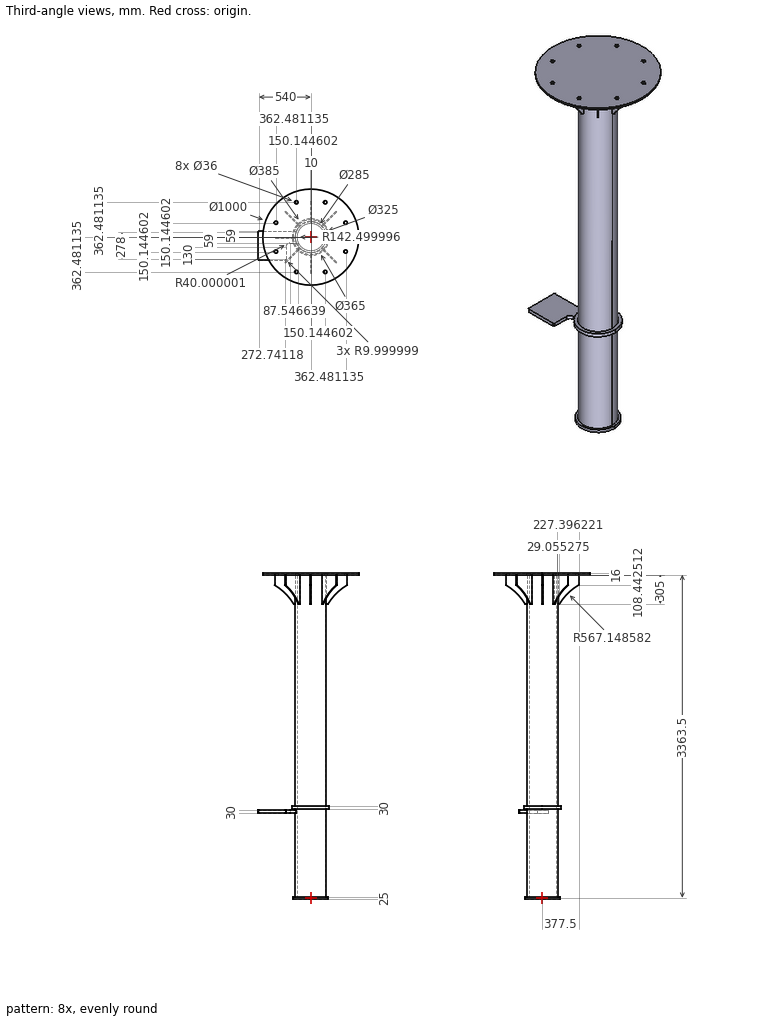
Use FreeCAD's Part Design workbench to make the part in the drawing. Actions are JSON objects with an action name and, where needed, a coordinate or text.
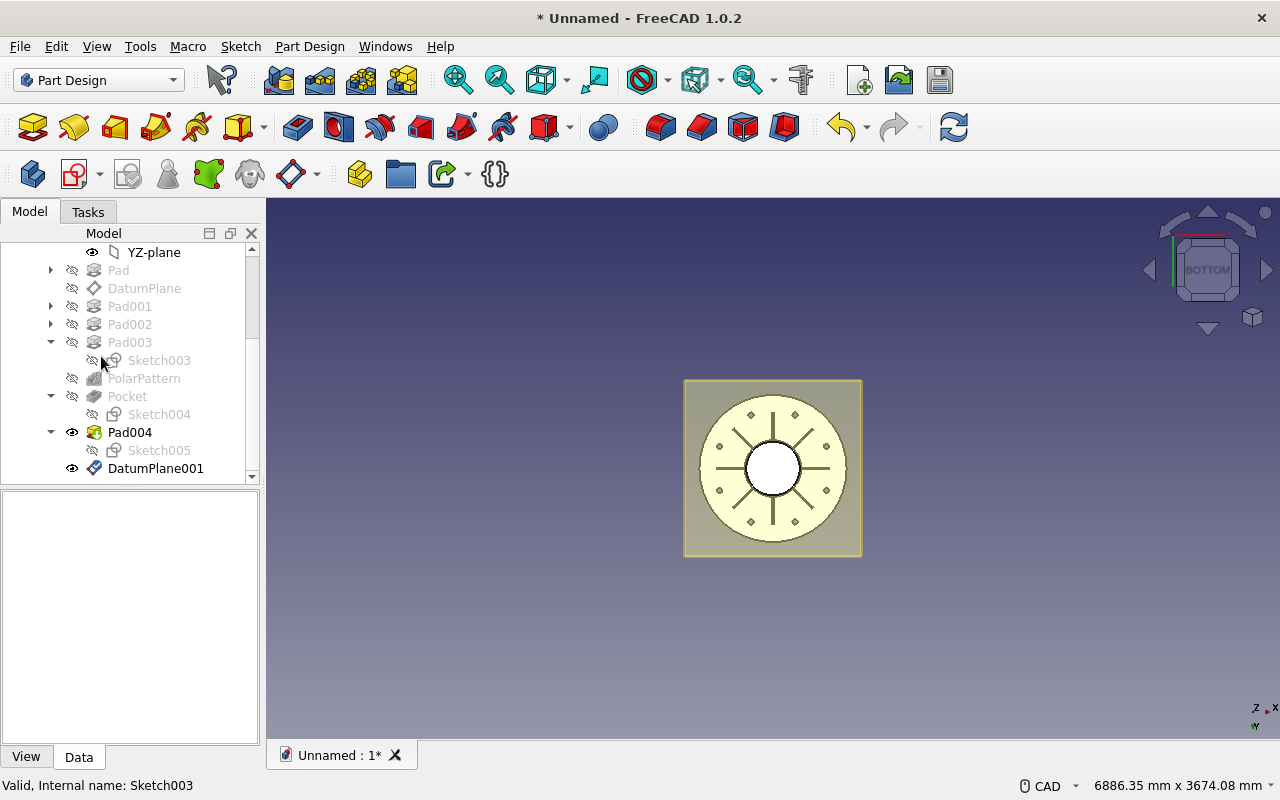
{"action": "left_click", "coordinate": [117, 468]}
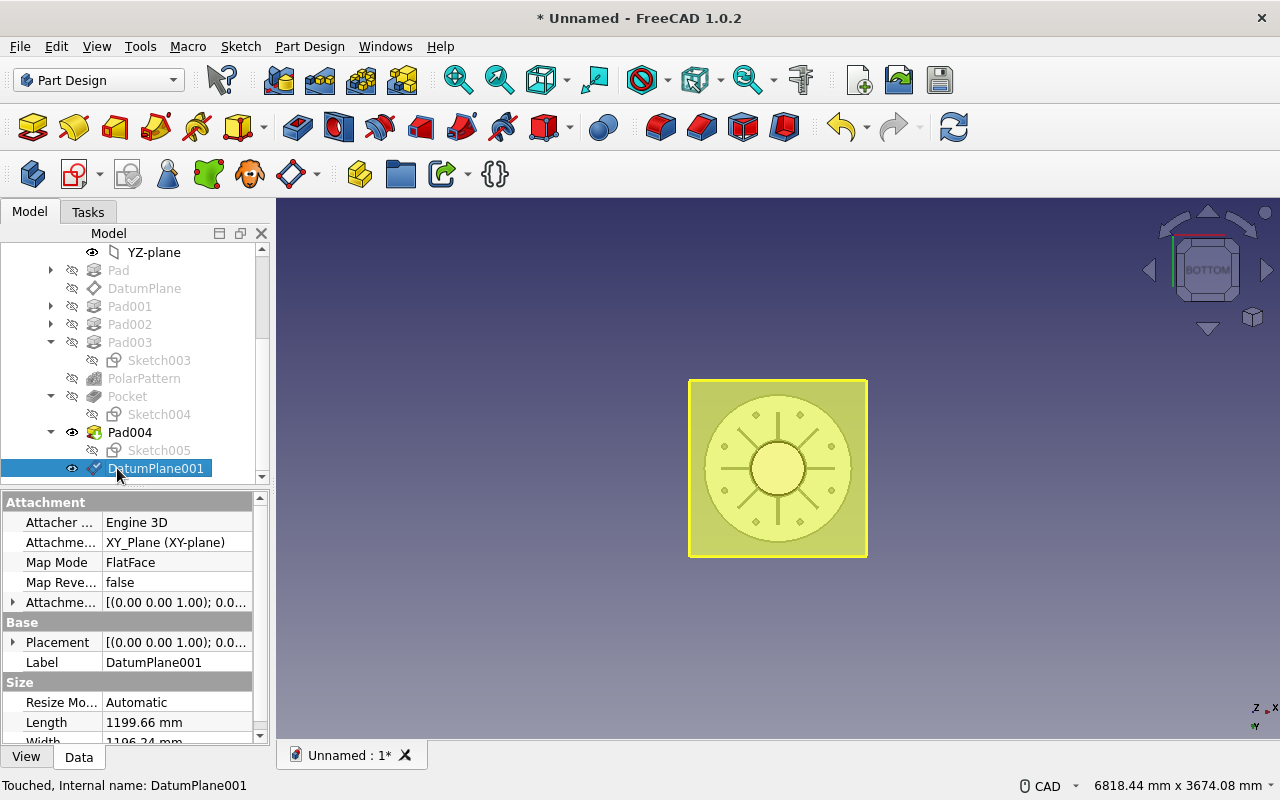
{"action": "left_click", "coordinate": [74, 174]}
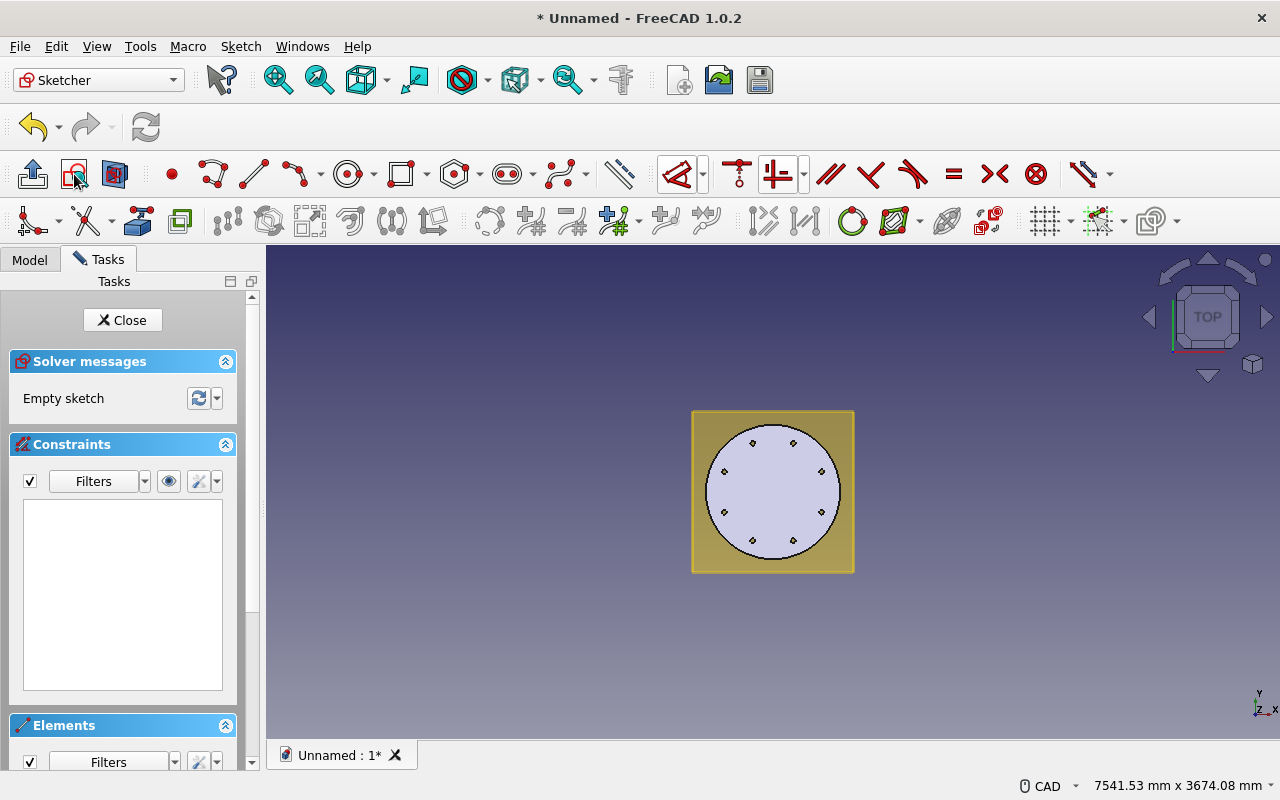
{"action": "left_click", "coordinate": [115, 174]}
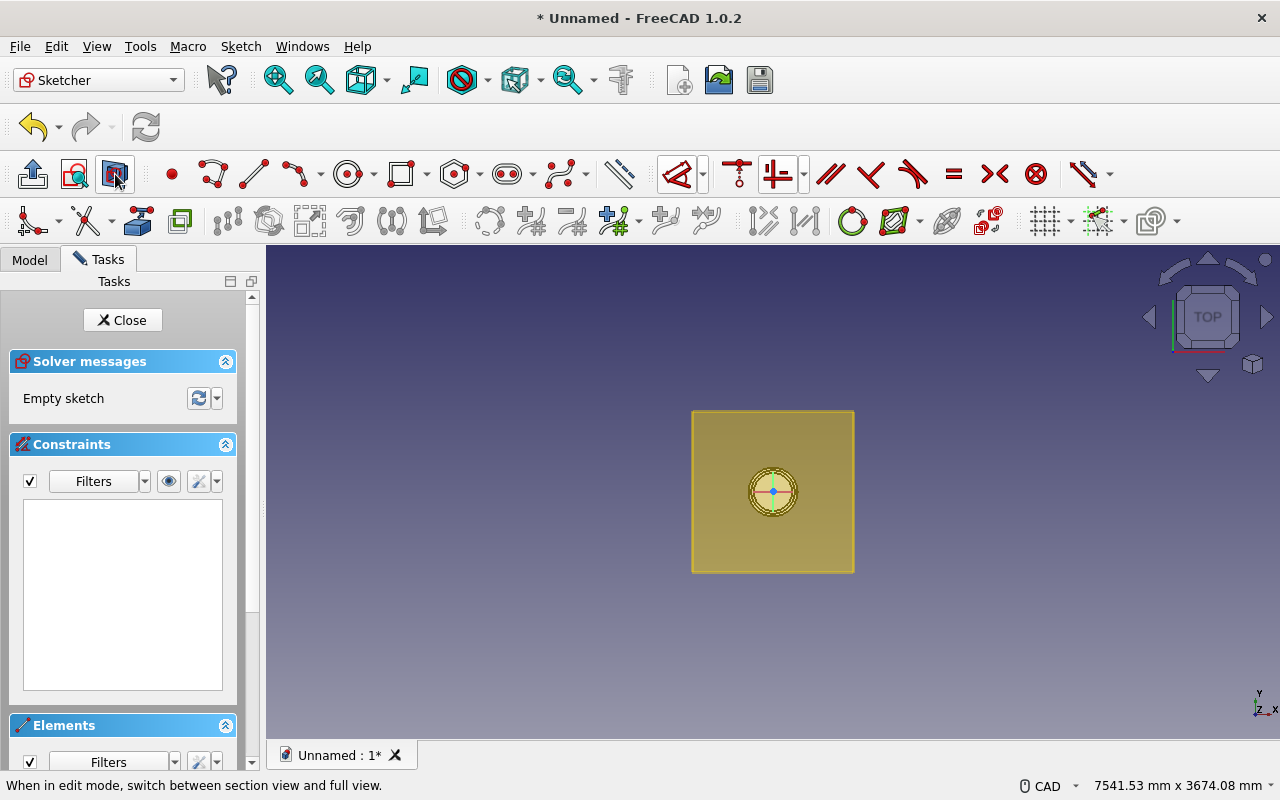
{"action": "scroll", "coordinate": [741, 506], "scroll_direction": "up", "scroll_amount": 10}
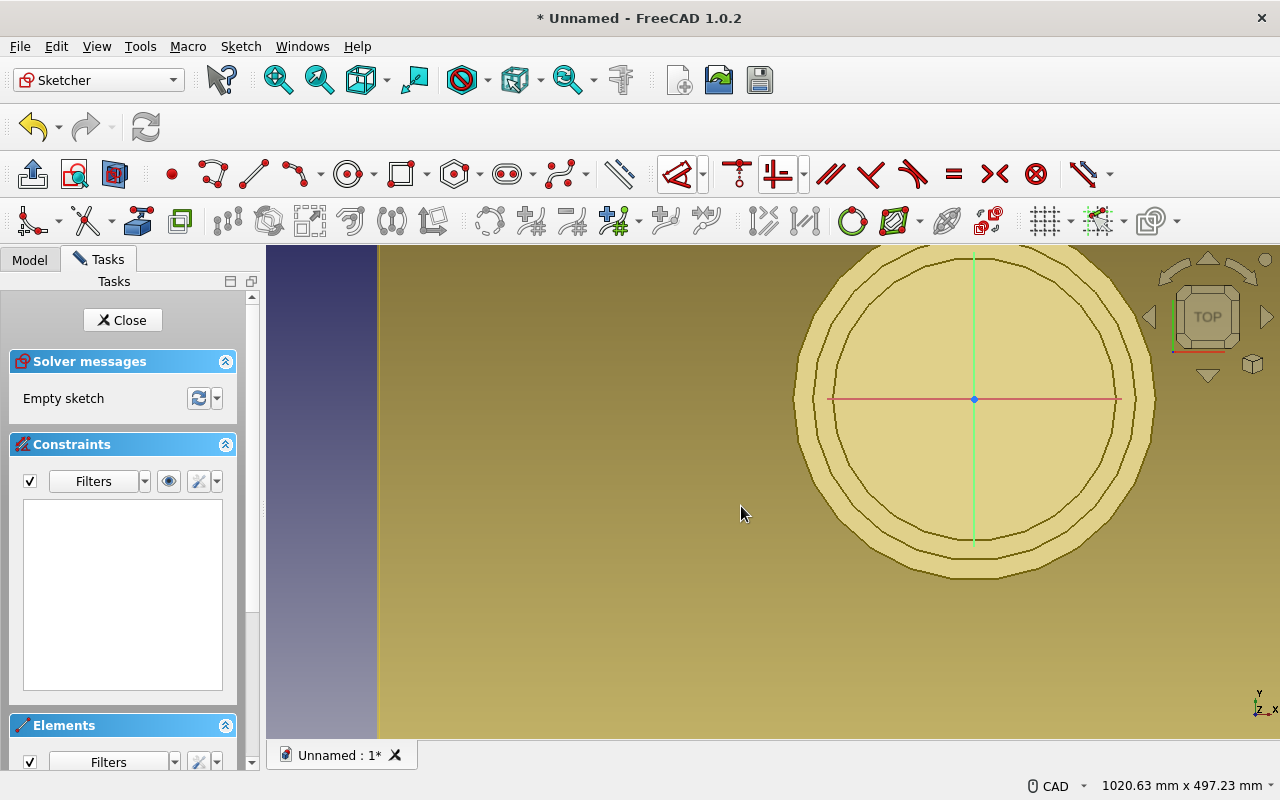
{"action": "key", "text": "g l"}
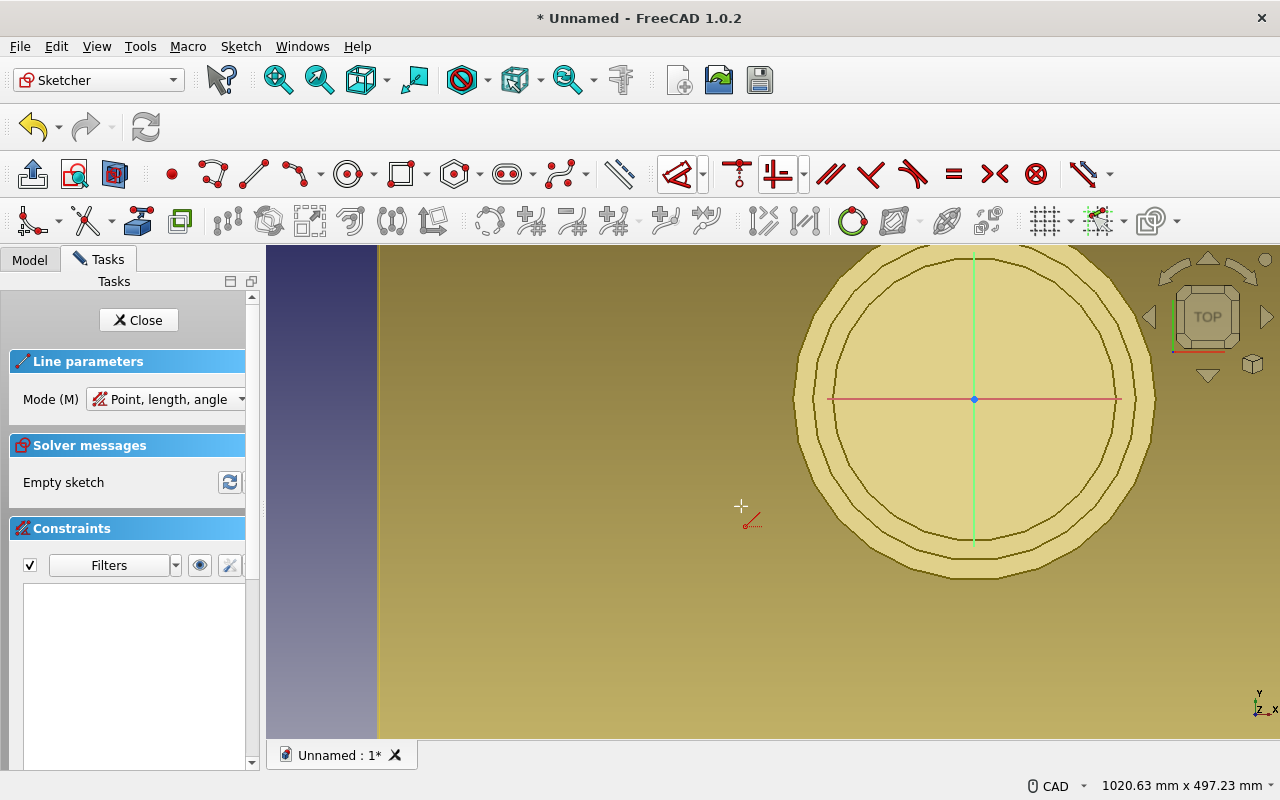
{"action": "left_click", "coordinate": [438, 341]}
{"action": "left_click", "coordinate": [846, 341]}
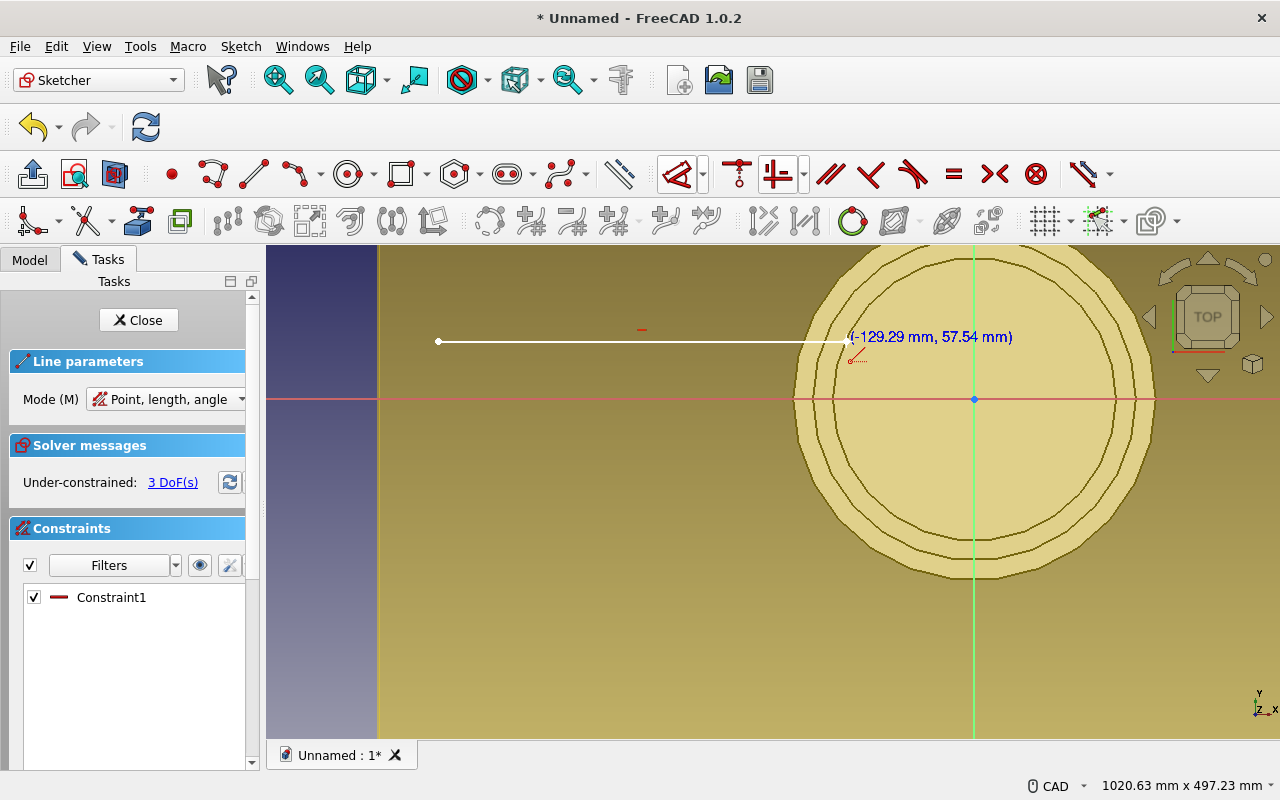
{"action": "left_click", "coordinate": [846, 458]}
{"action": "left_click", "coordinate": [759, 458]}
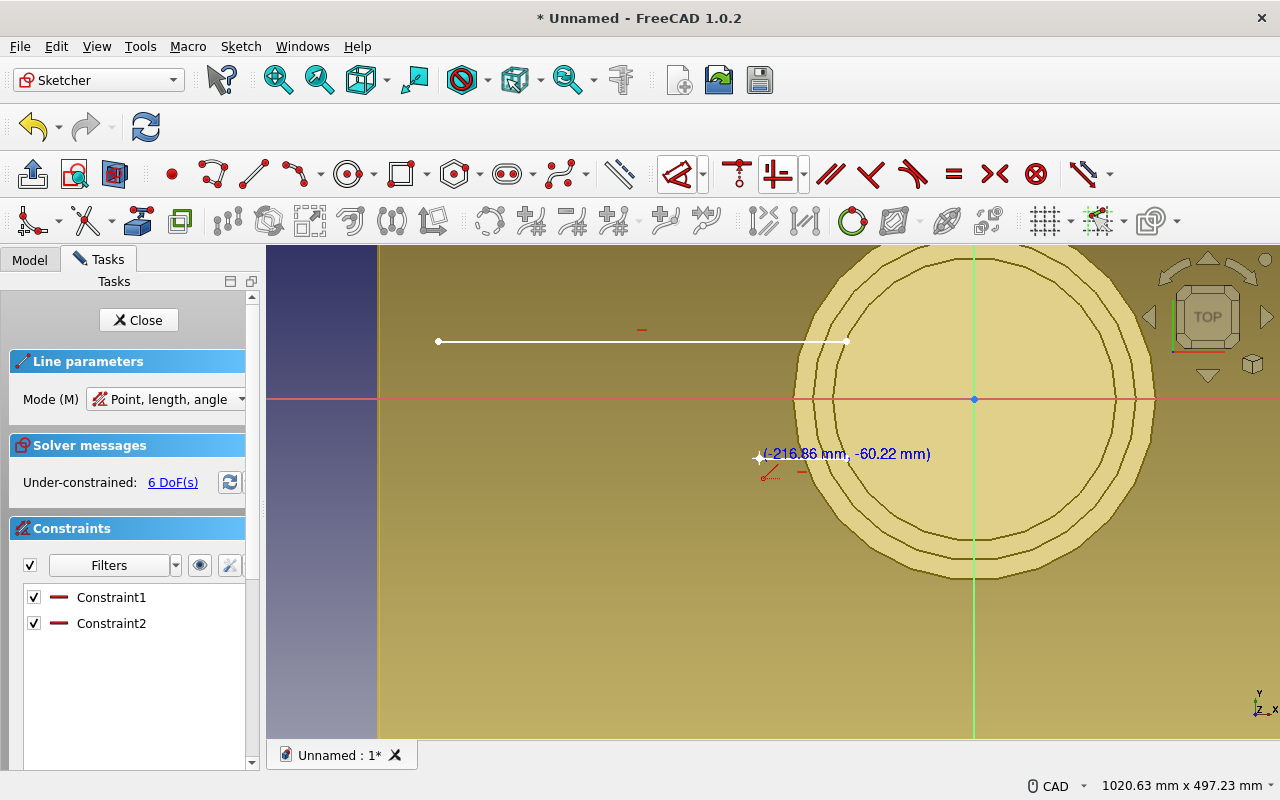
{"action": "left_click", "coordinate": [719, 498]}
{"action": "left_click", "coordinate": [719, 627]}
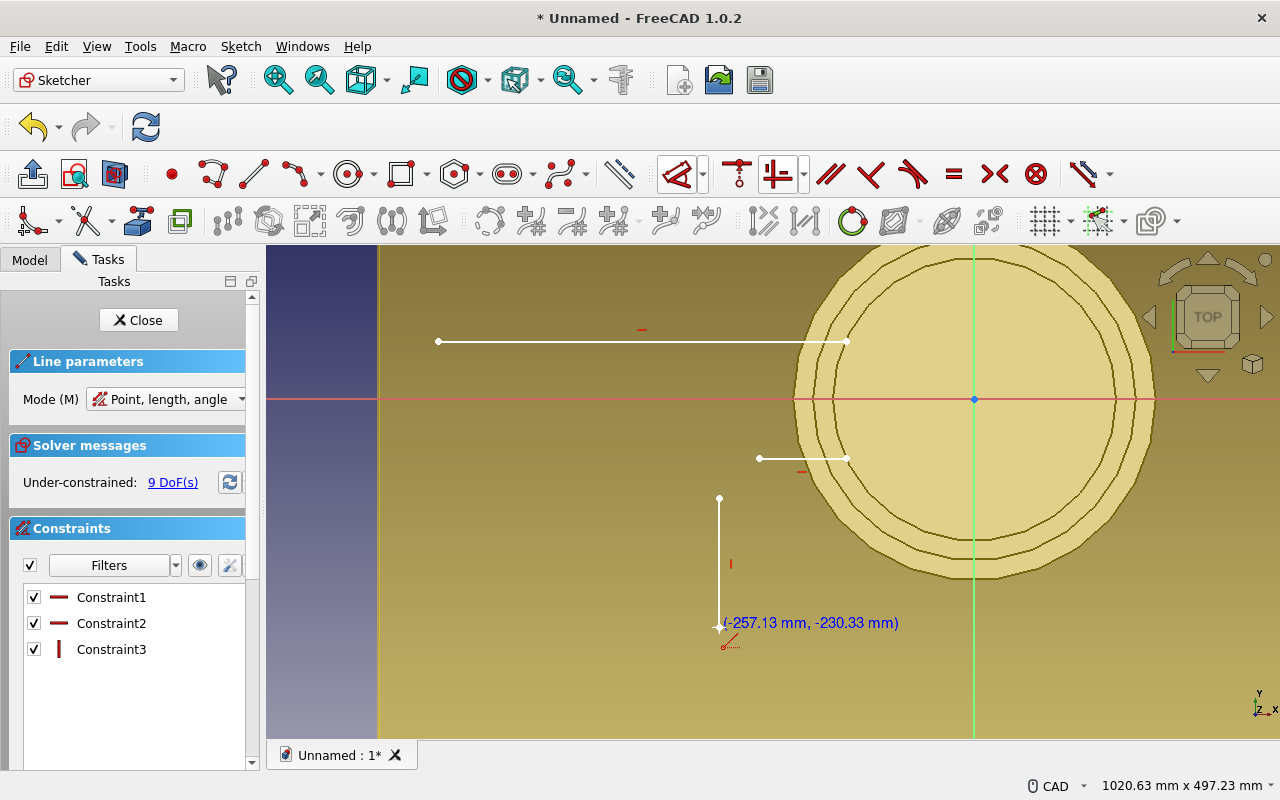
{"action": "left_click", "coordinate": [709, 637]}
{"action": "left_click", "coordinate": [438, 637]}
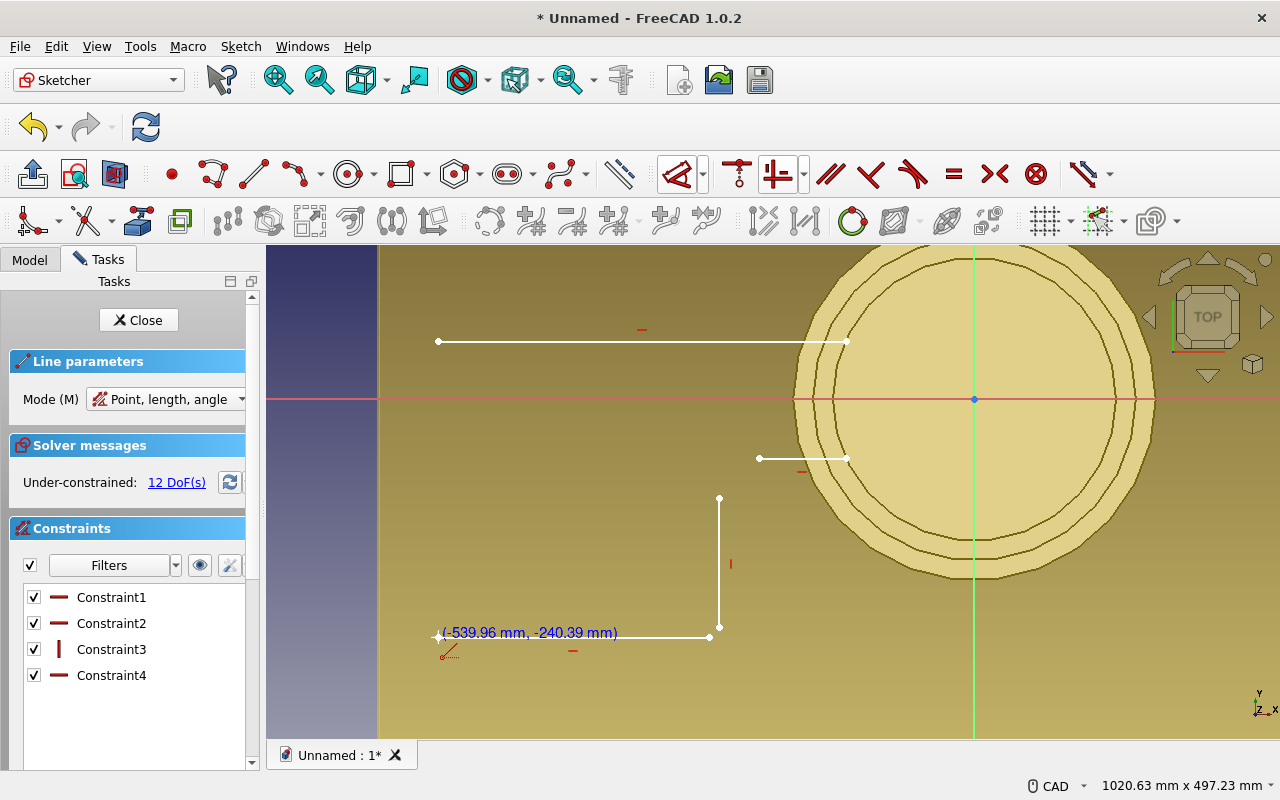
{"action": "left_click", "coordinate": [428, 627]}
{"action": "left_click", "coordinate": [428, 350]}